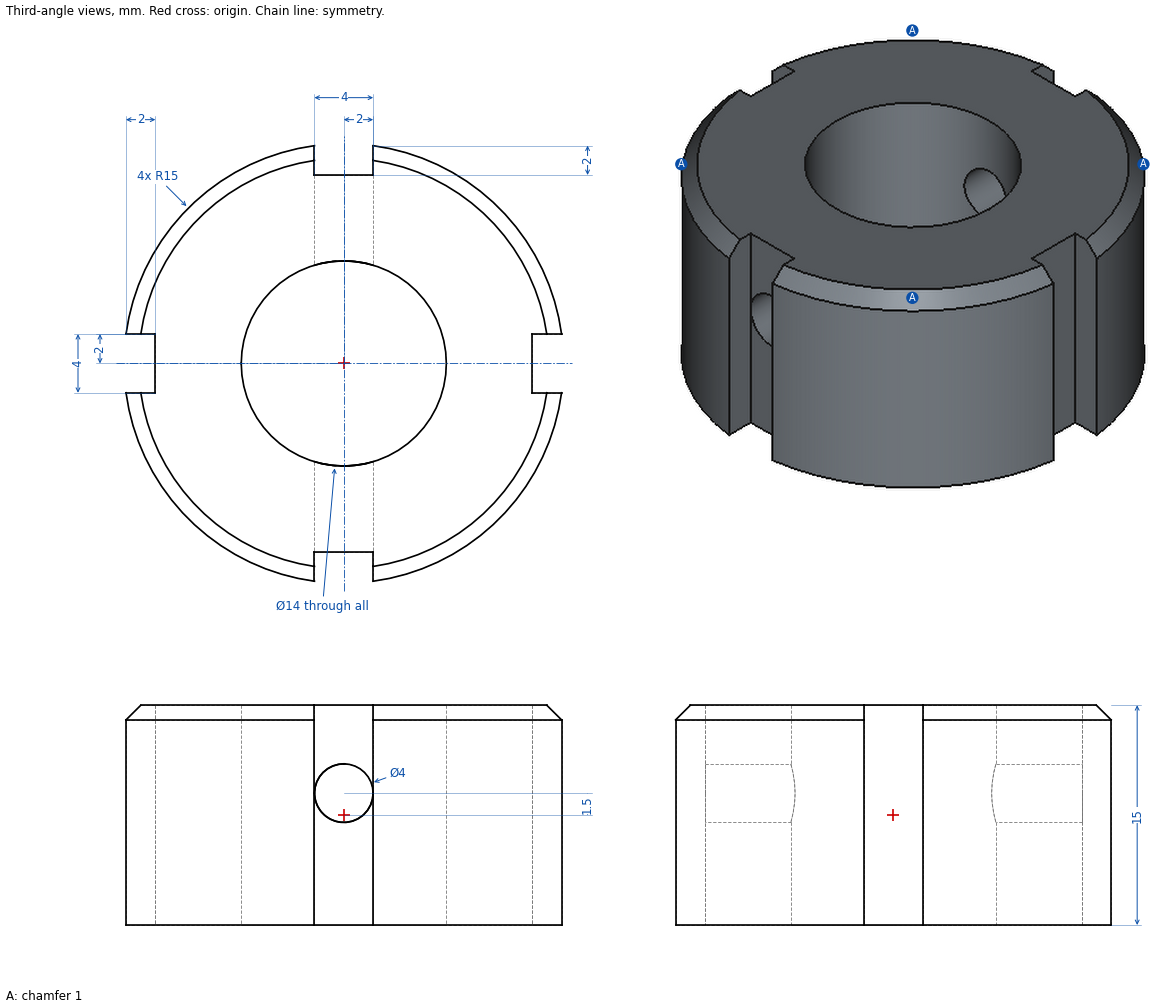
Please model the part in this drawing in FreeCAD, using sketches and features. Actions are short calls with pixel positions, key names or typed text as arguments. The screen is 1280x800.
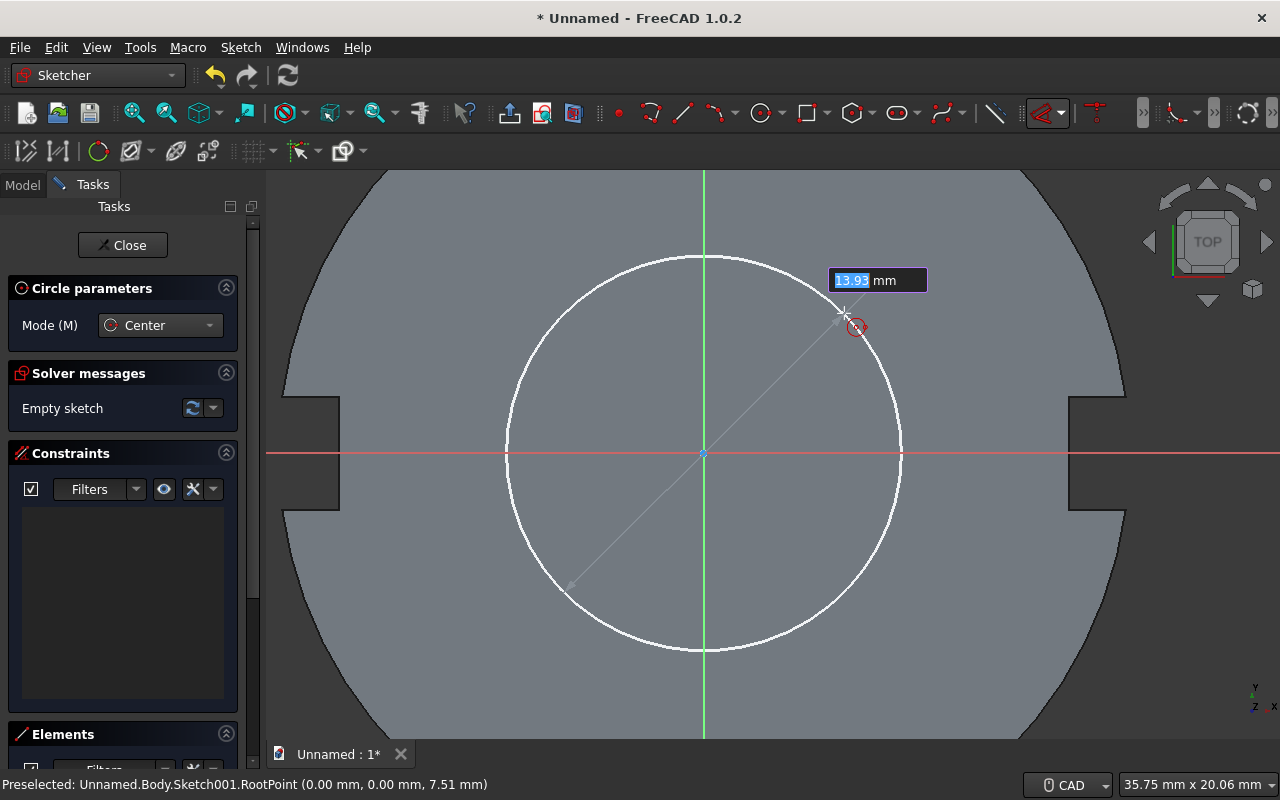
text(14)
key(Return)
key(Escape)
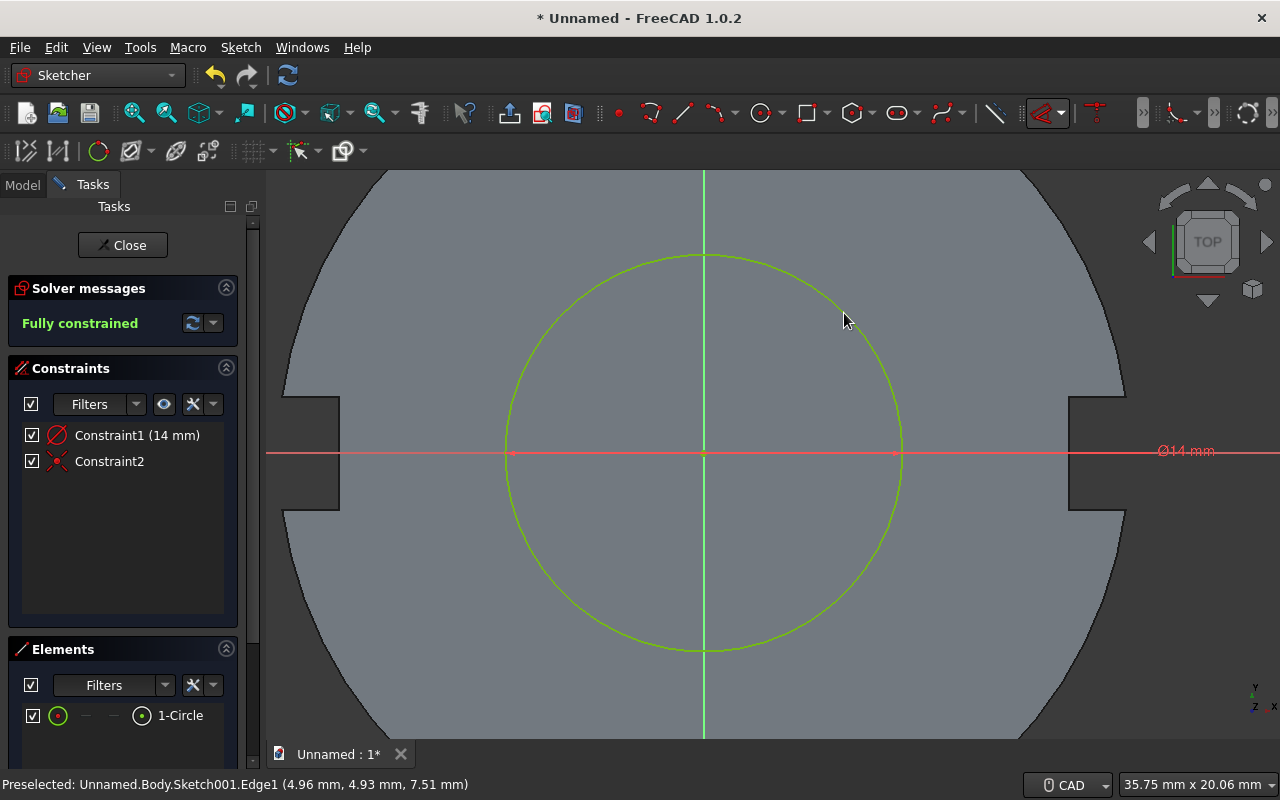
click(123, 245)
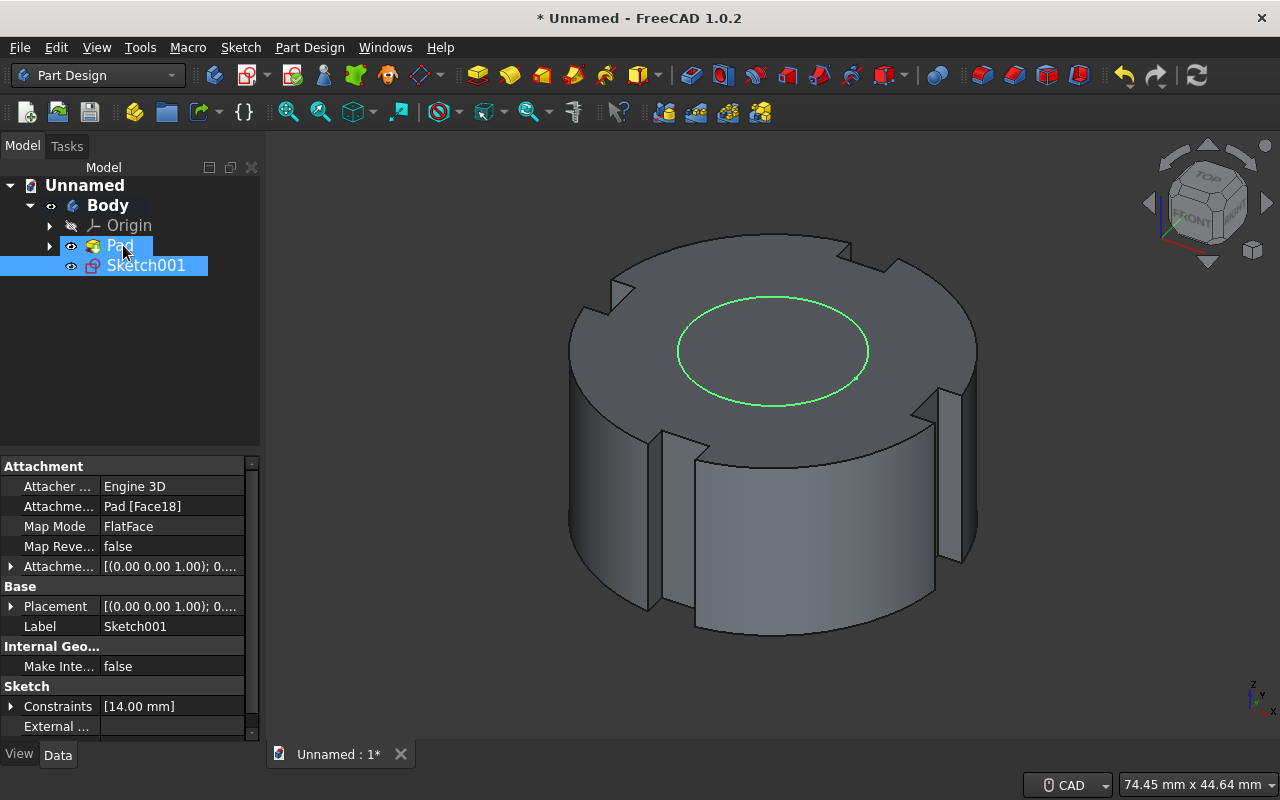
click(724, 76)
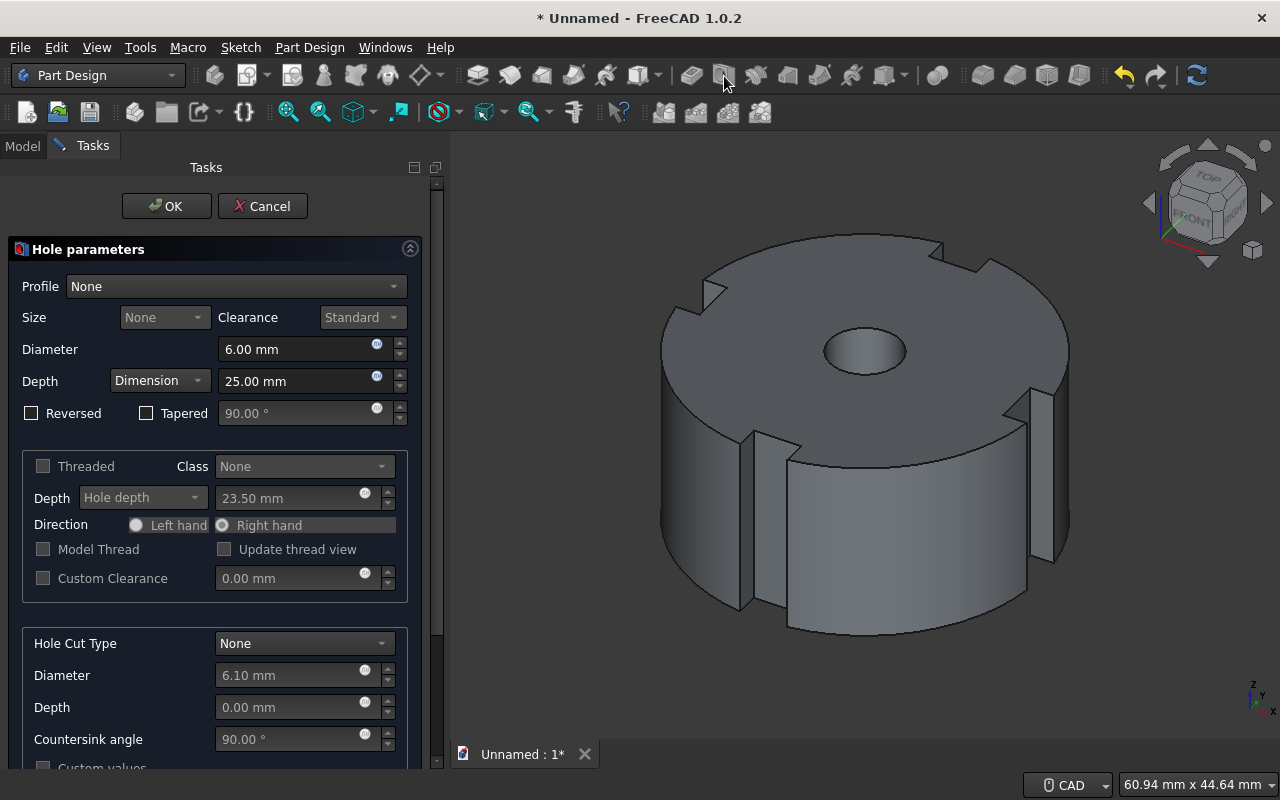
triple_click(305, 349)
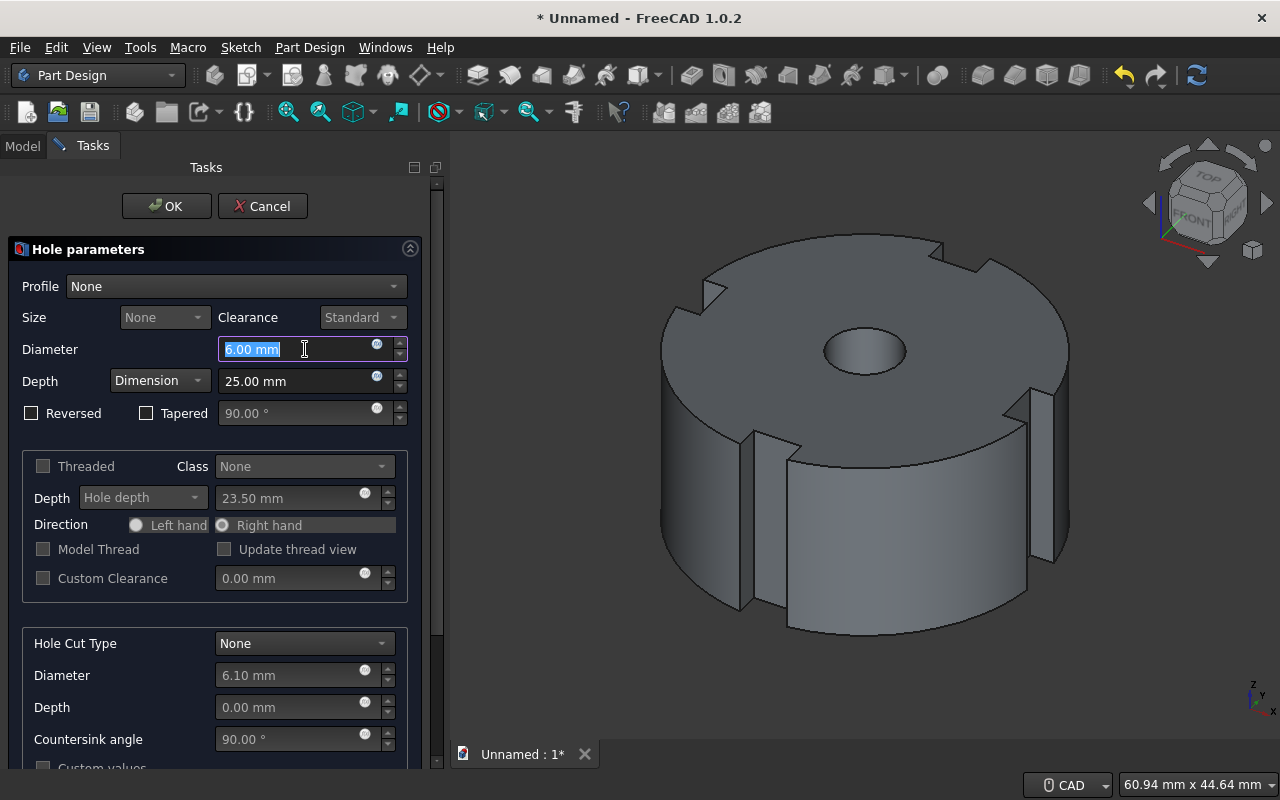
text(14)
key(Tab)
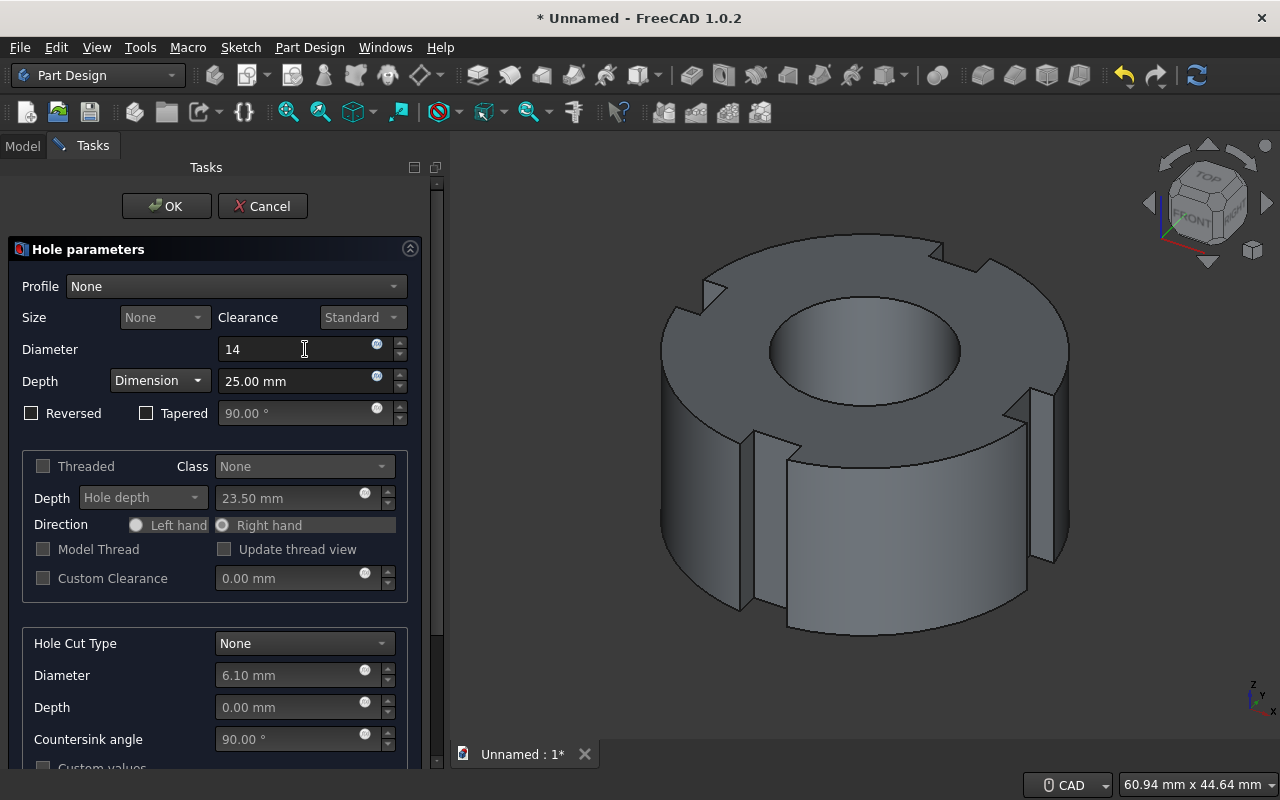
click(161, 380)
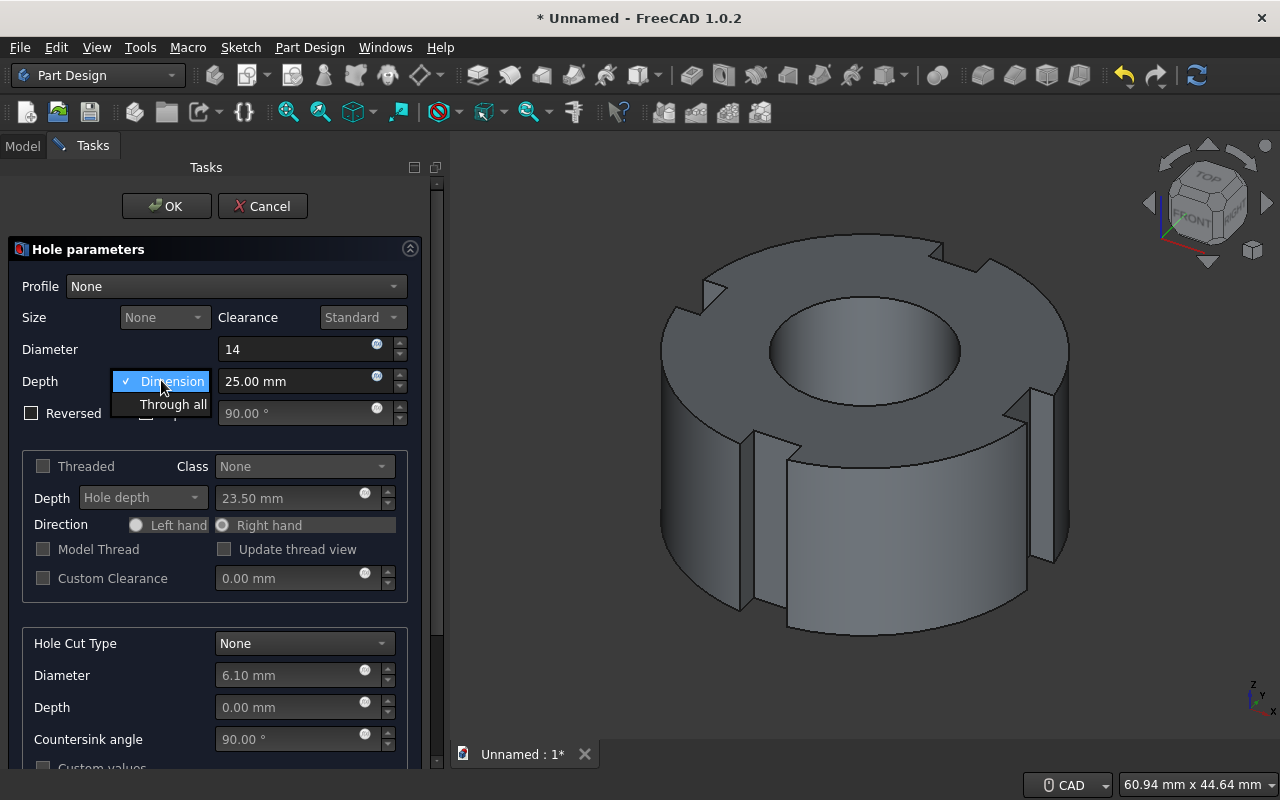
click(160, 404)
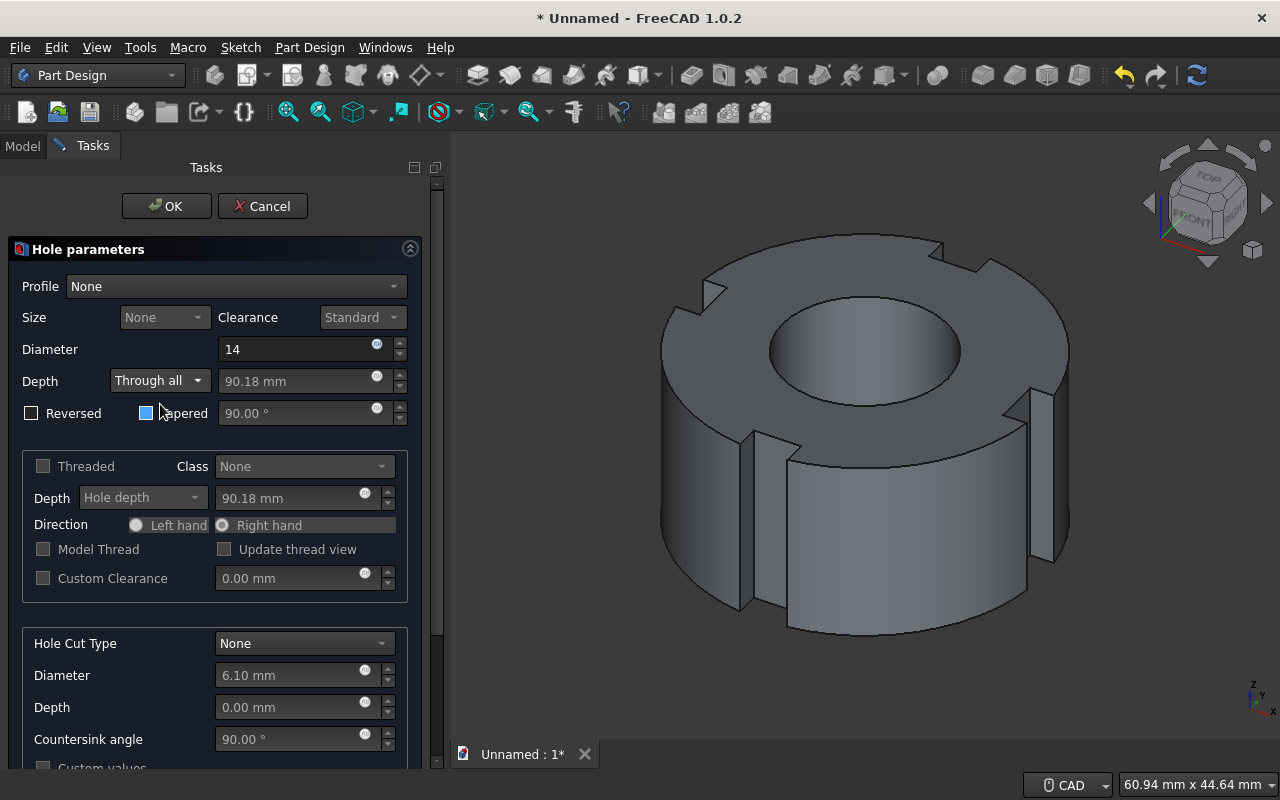
click(167, 206)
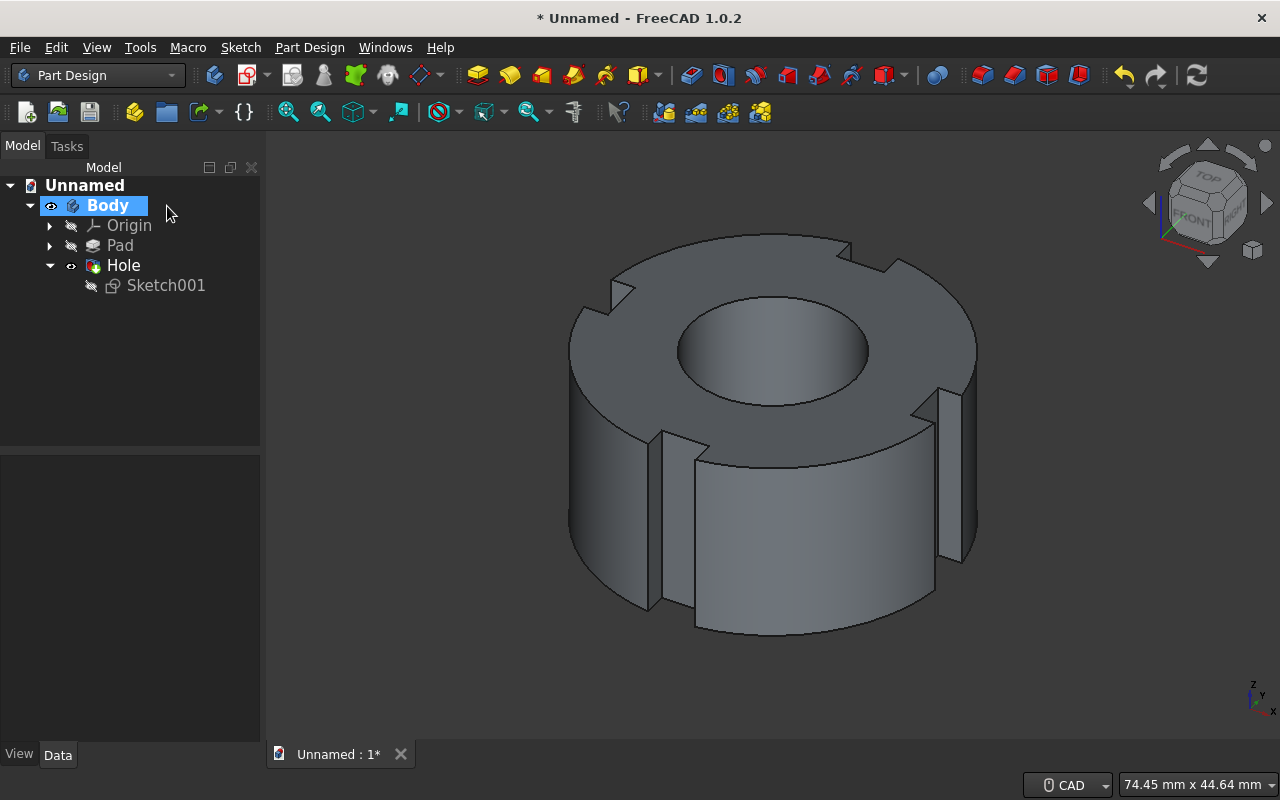
click(576, 381)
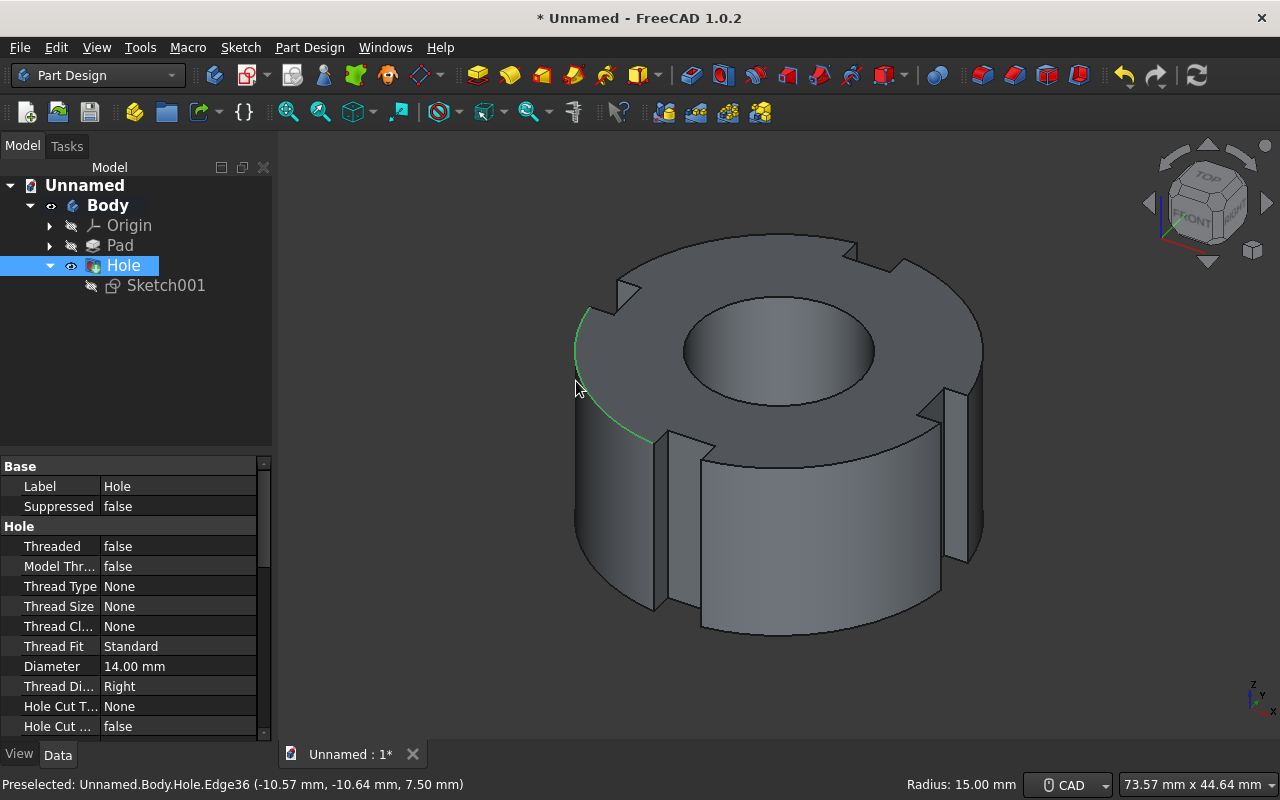
click(832, 464, ctrl)